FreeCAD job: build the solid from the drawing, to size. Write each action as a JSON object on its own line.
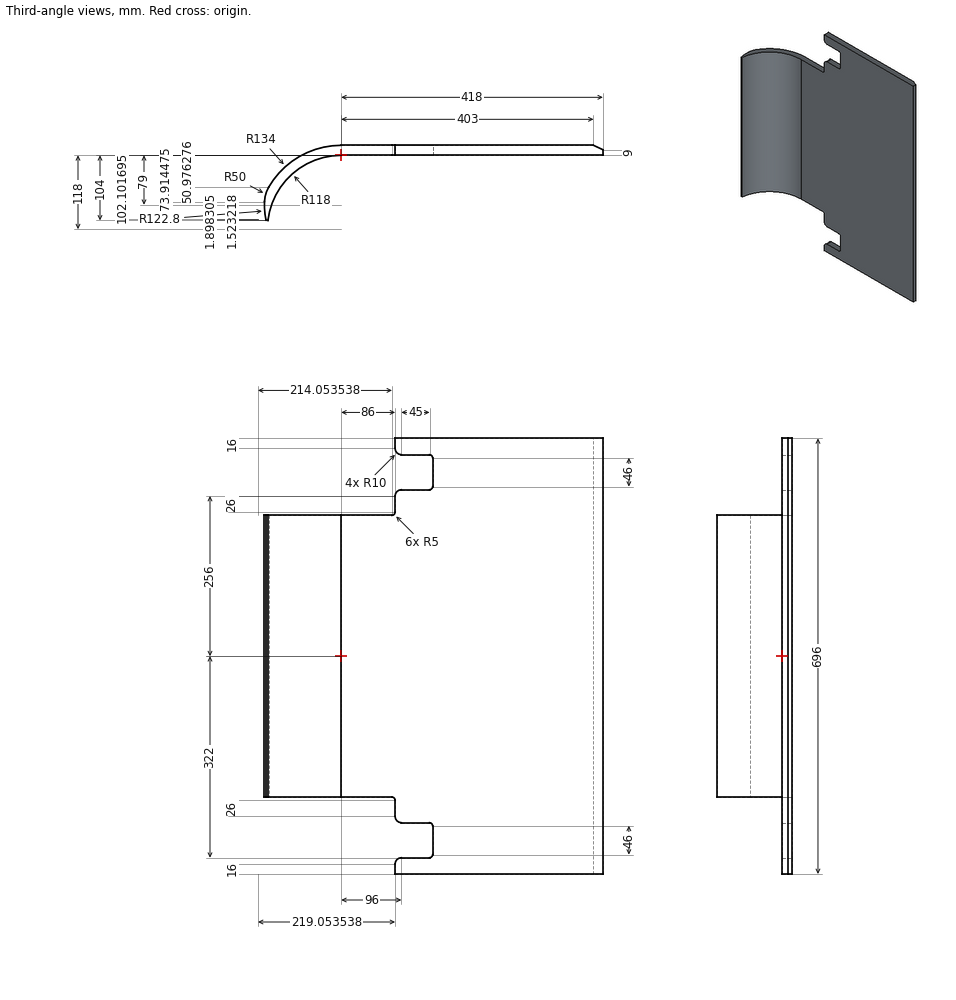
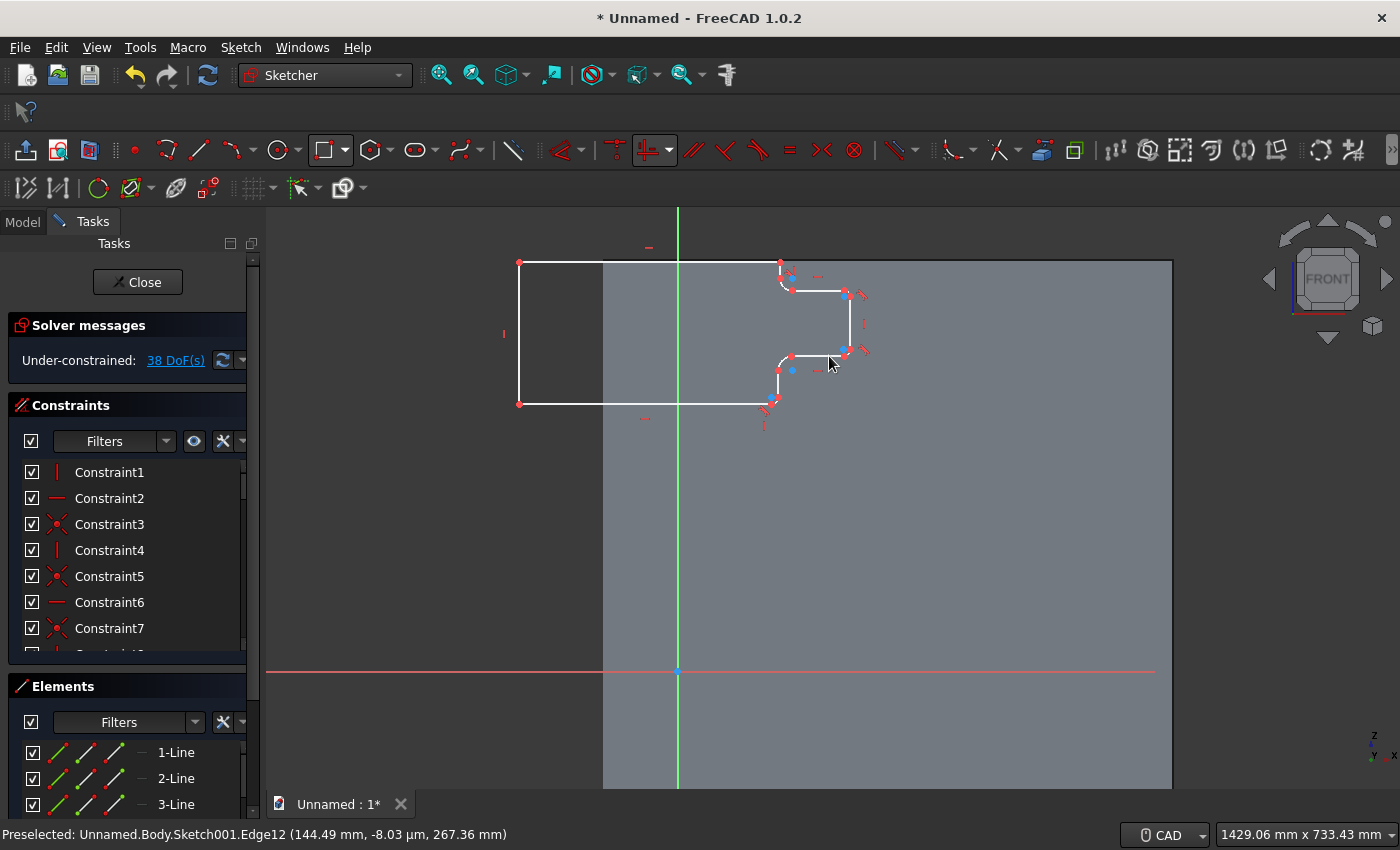
{"action": "left_click", "coordinate": [829, 356]}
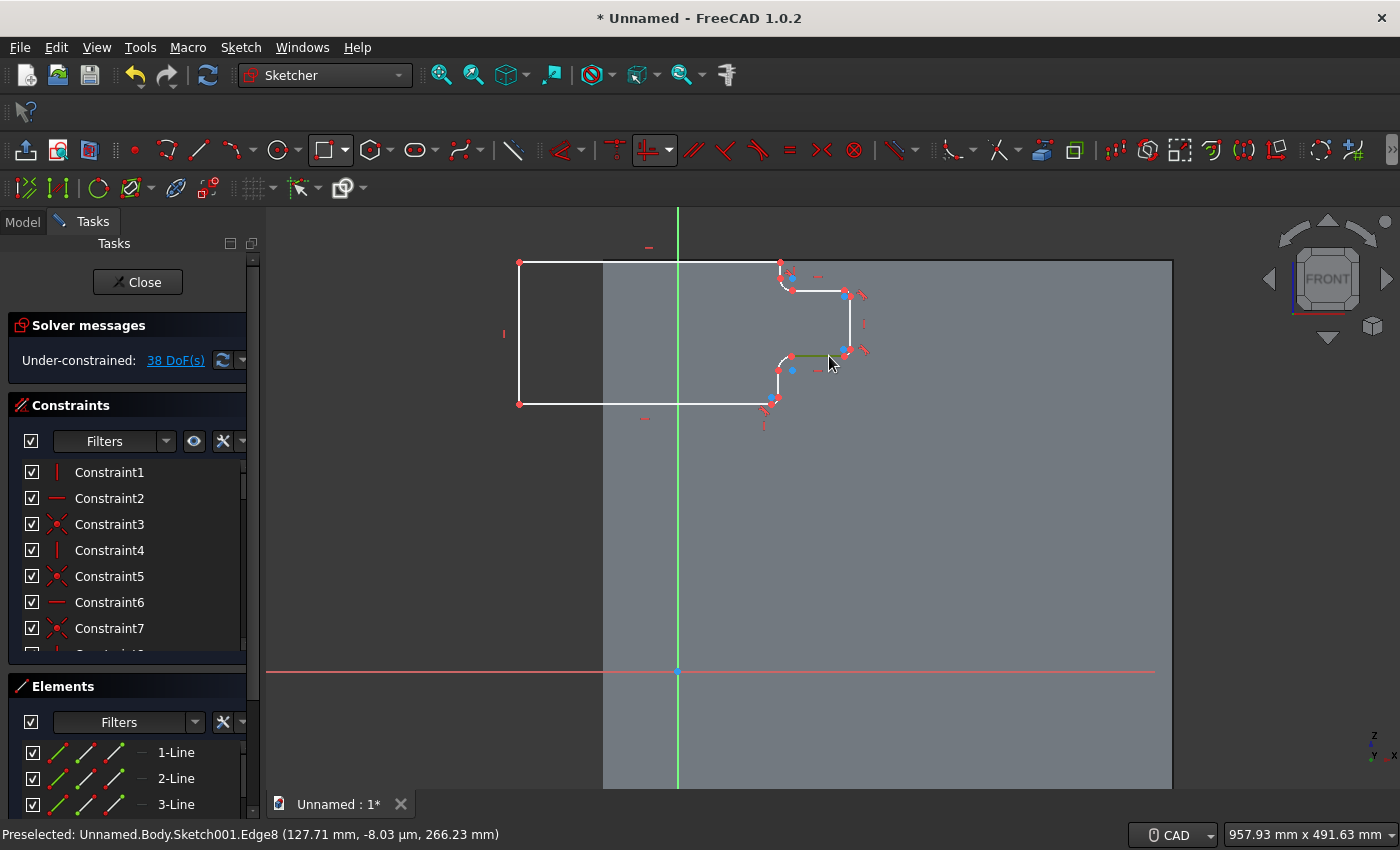
{"action": "scroll", "coordinate": [849, 354], "scroll_direction": "up", "scroll_amount": 6}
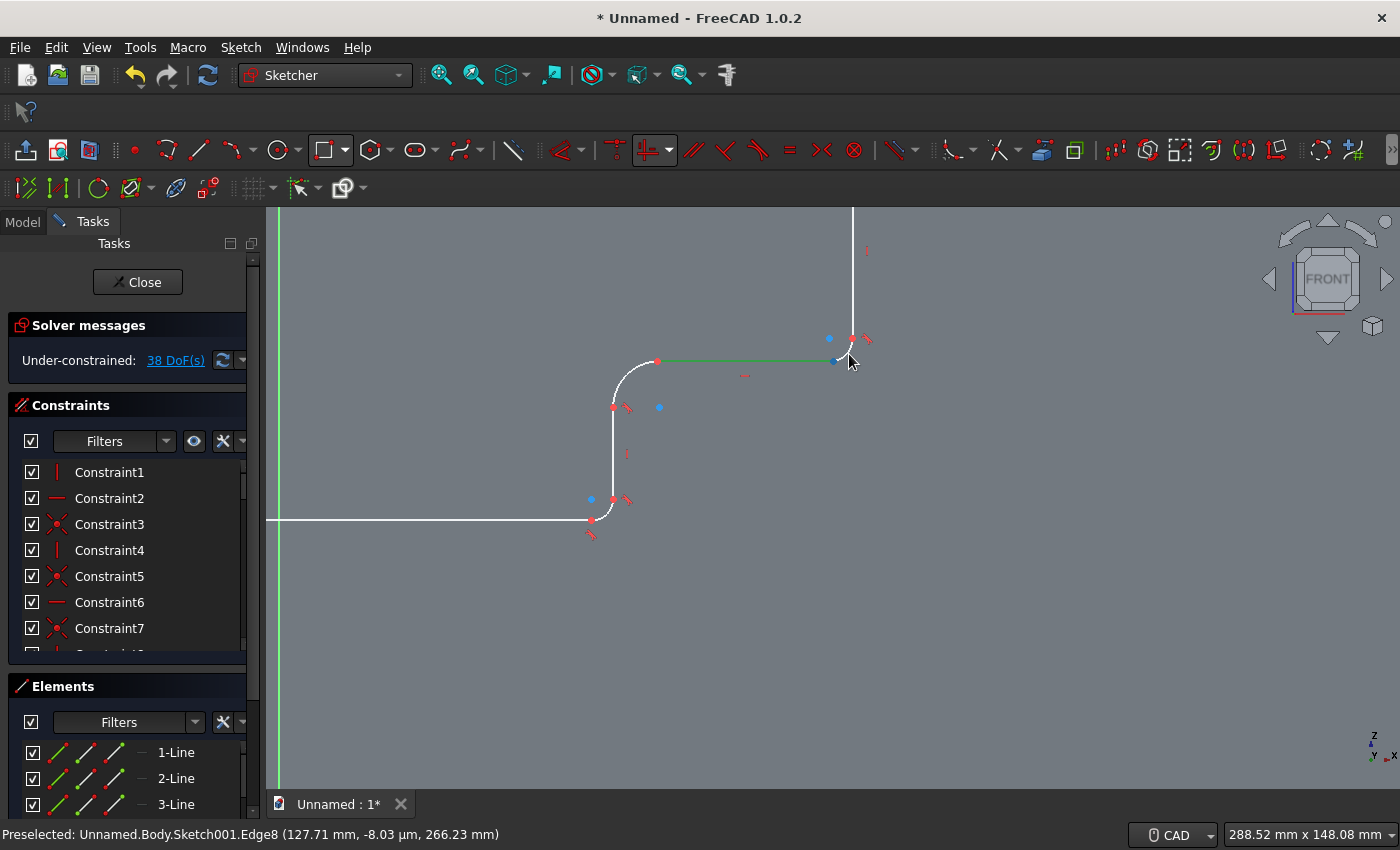
{"action": "left_click", "coordinate": [847, 354]}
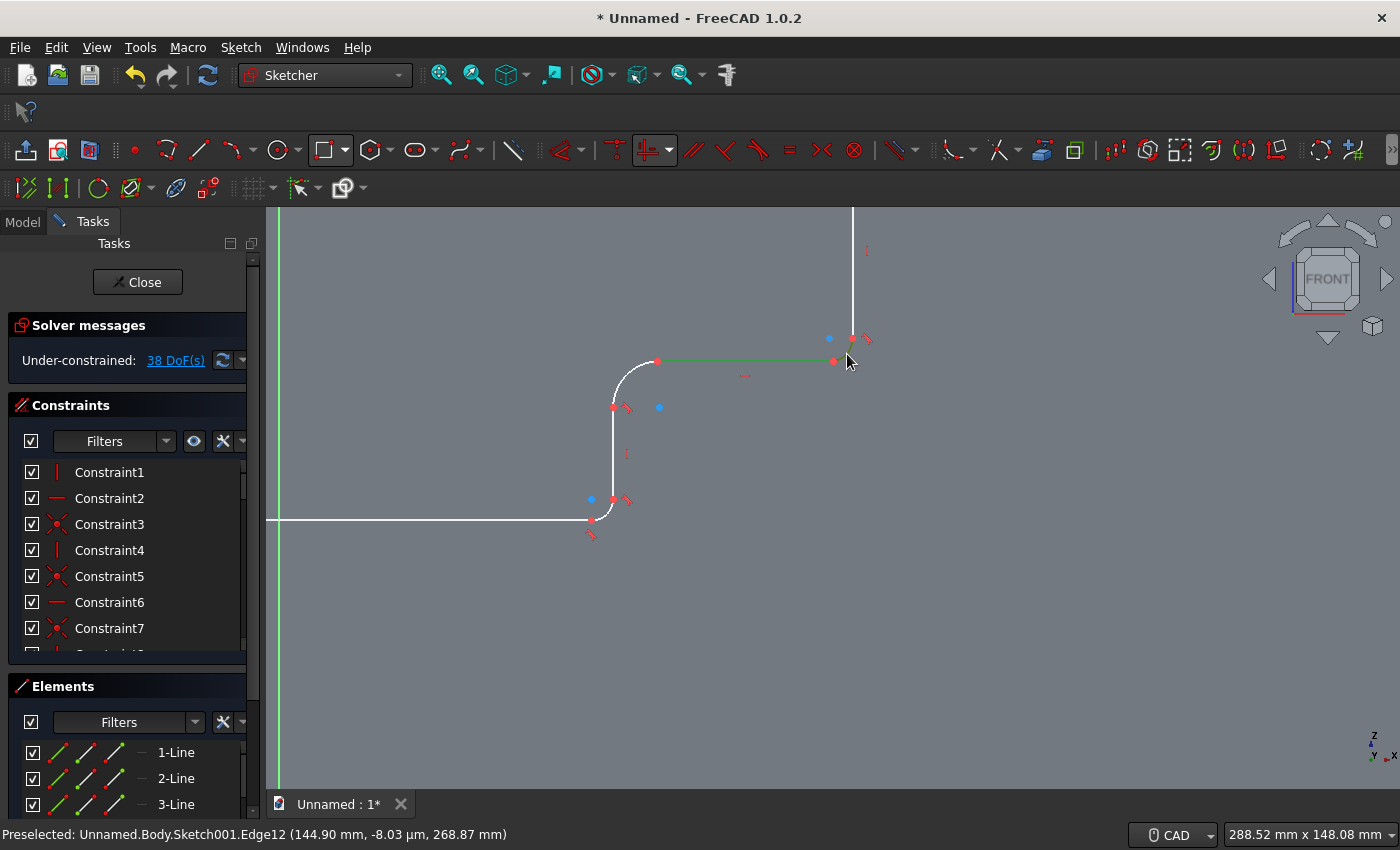
{"action": "left_click", "coordinate": [758, 150]}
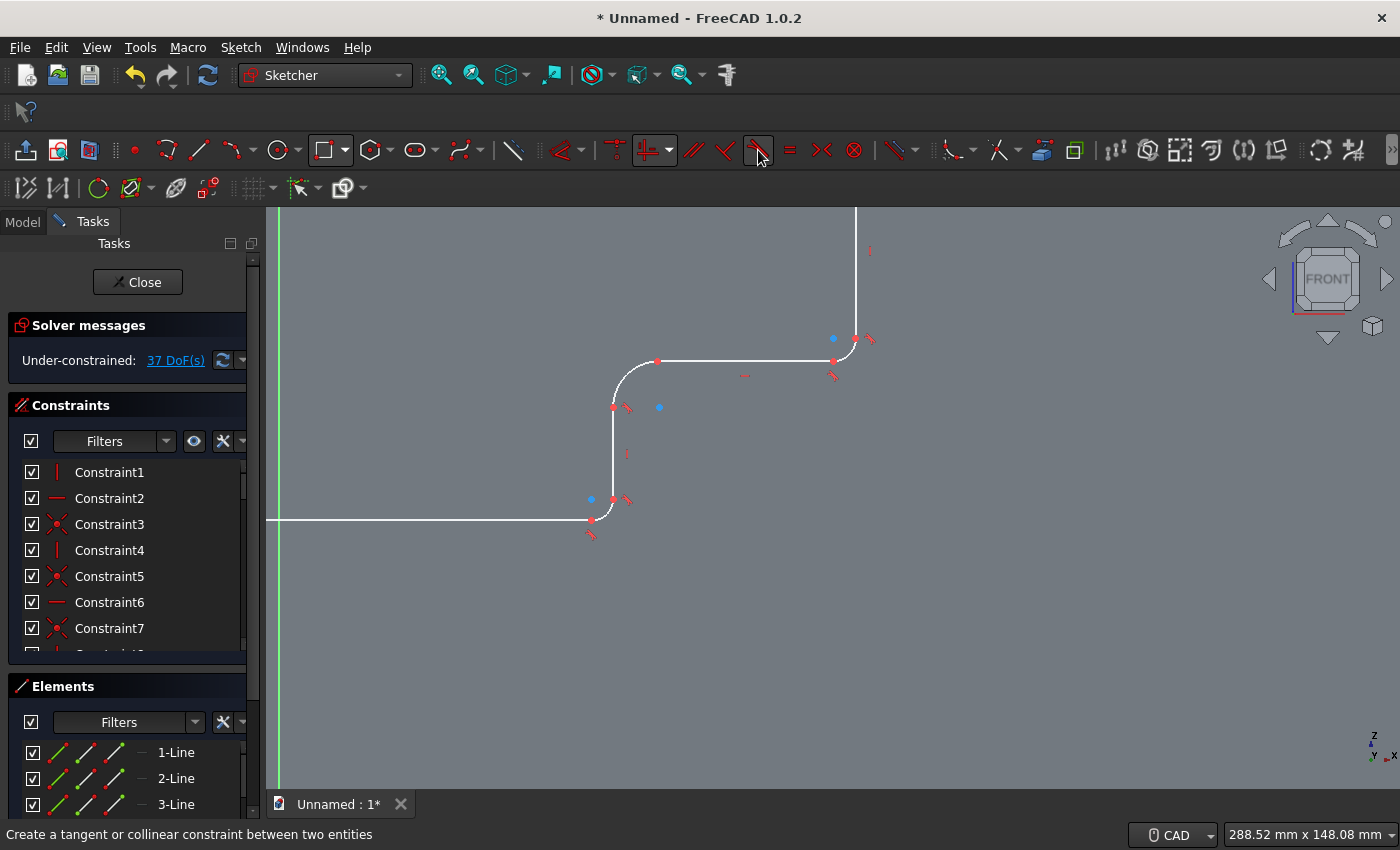
{"action": "scroll", "coordinate": [836, 356], "scroll_direction": "down", "scroll_amount": 10}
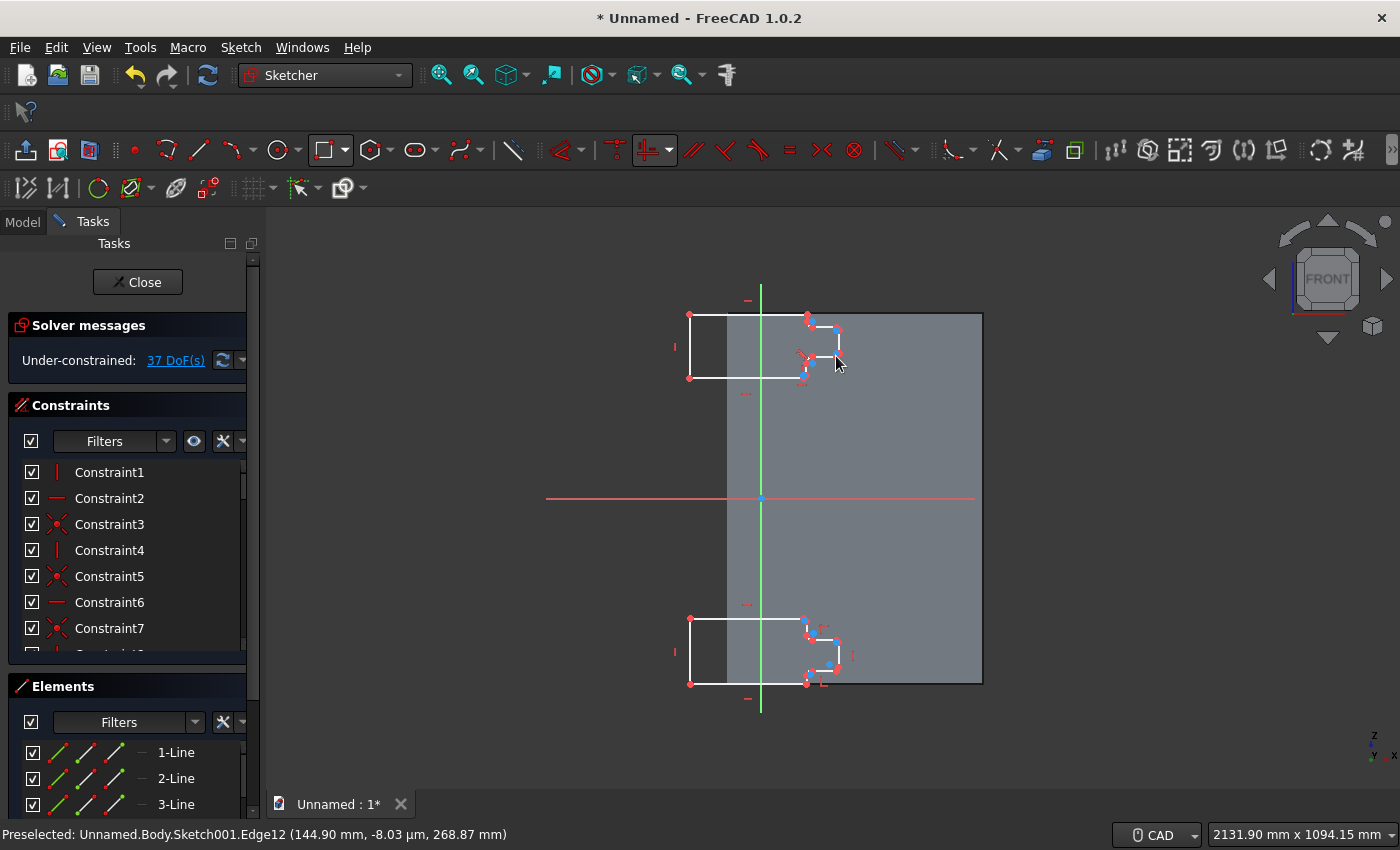
{"action": "scroll", "coordinate": [829, 357], "scroll_direction": "up", "scroll_amount": 4}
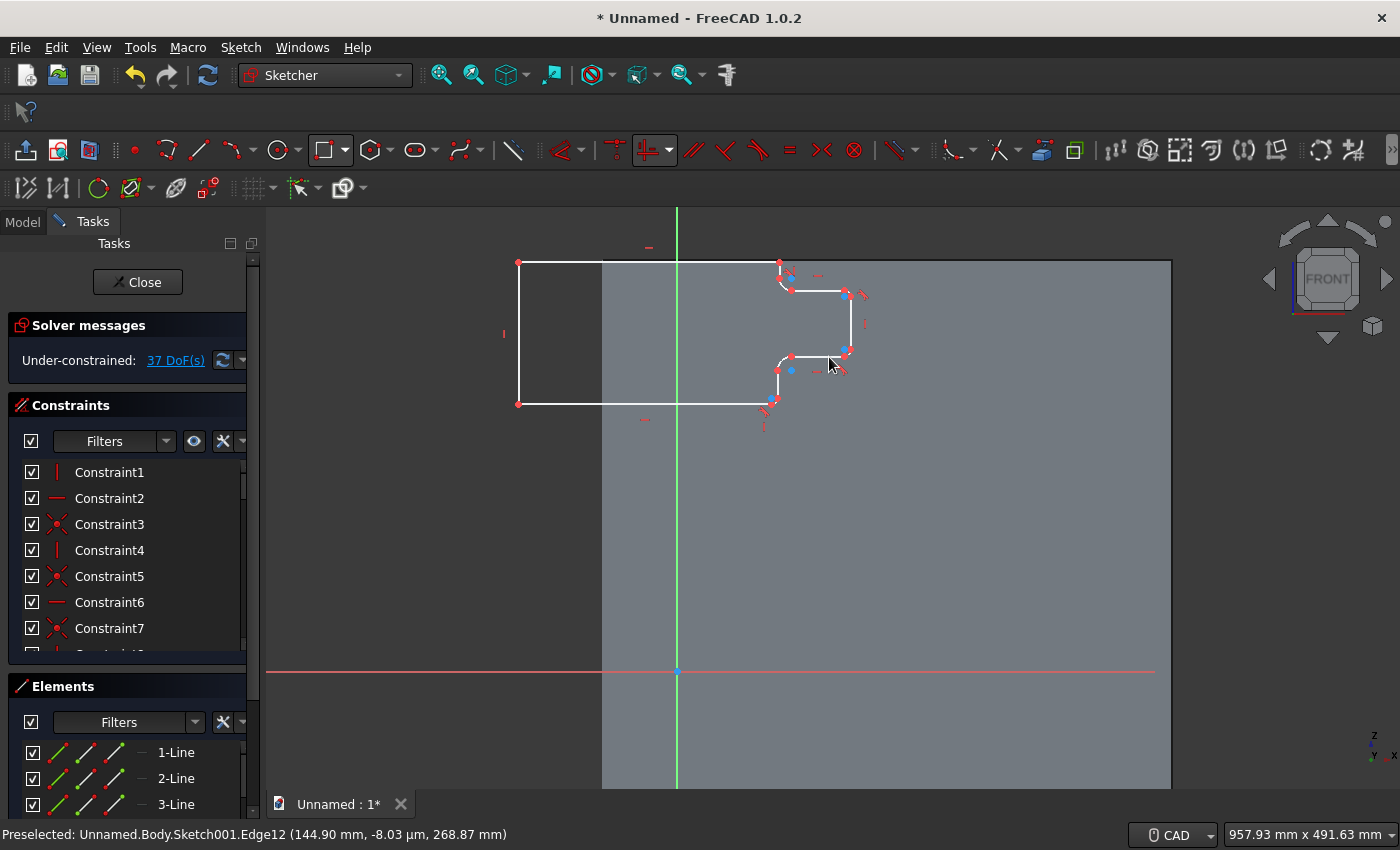
{"action": "left_click", "coordinate": [828, 357]}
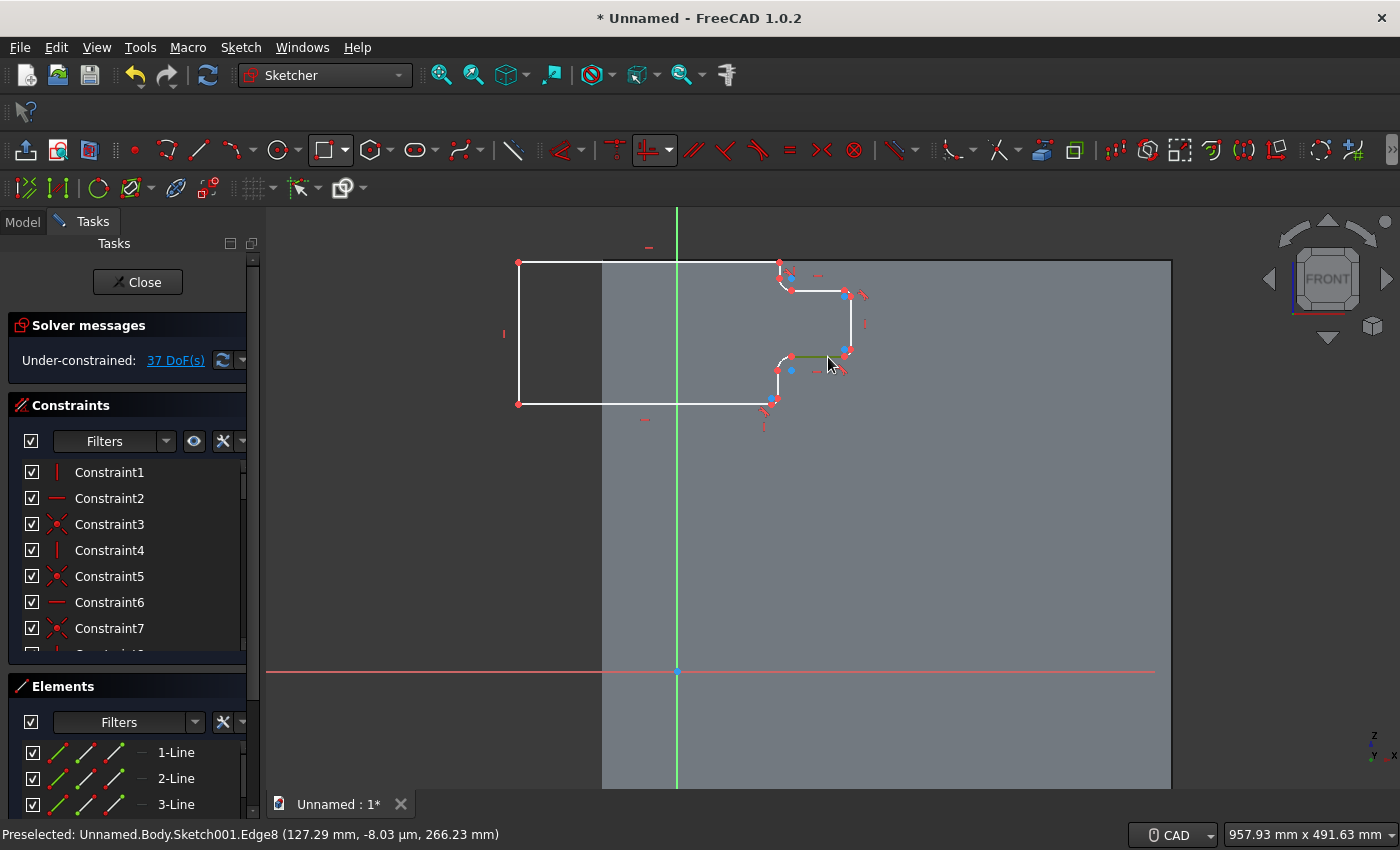
{"action": "scroll", "coordinate": [782, 361], "scroll_direction": "up", "scroll_amount": 2}